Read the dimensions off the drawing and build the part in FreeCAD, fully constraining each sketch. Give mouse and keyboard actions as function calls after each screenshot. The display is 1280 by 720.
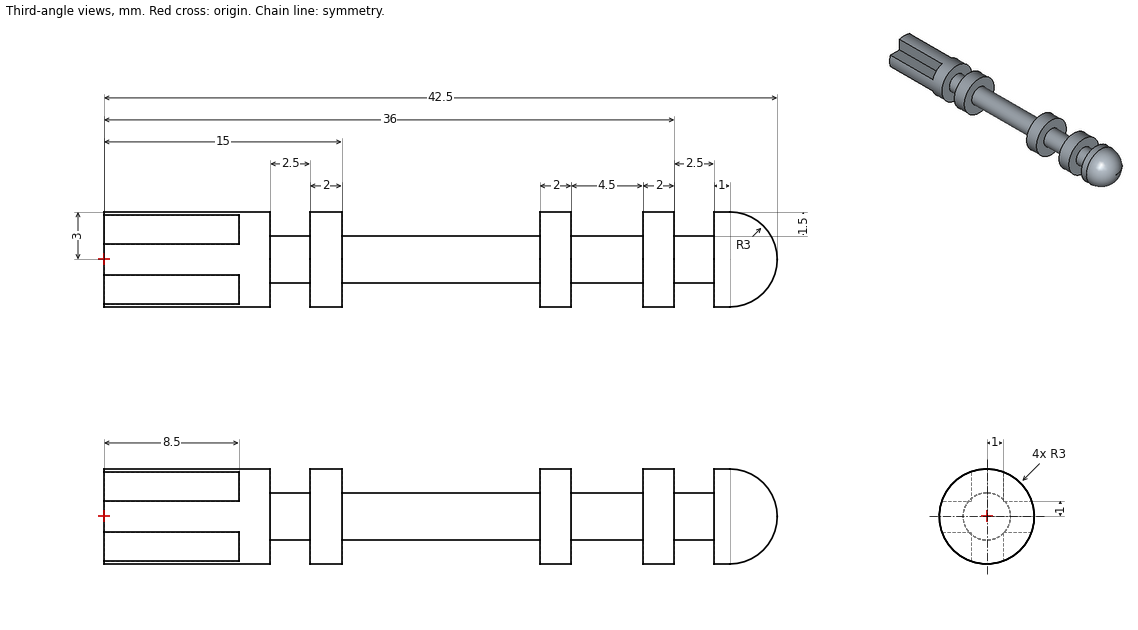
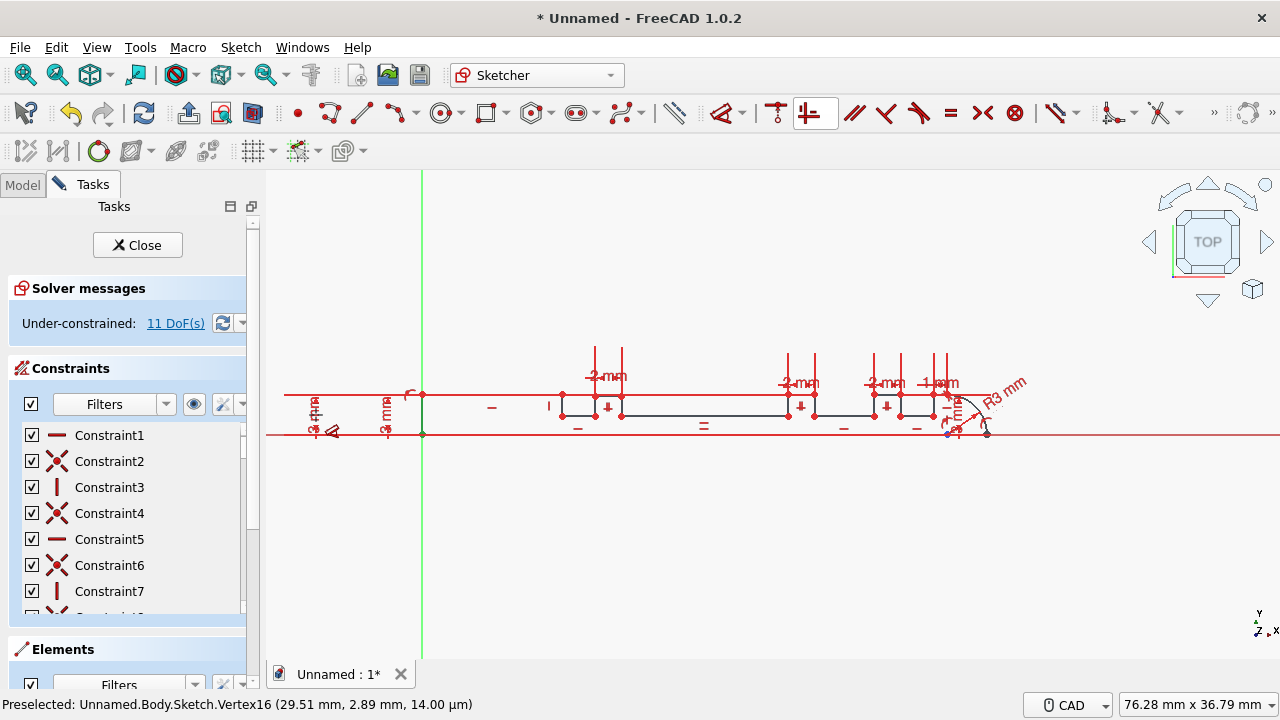
click(622, 396)
click(656, 402)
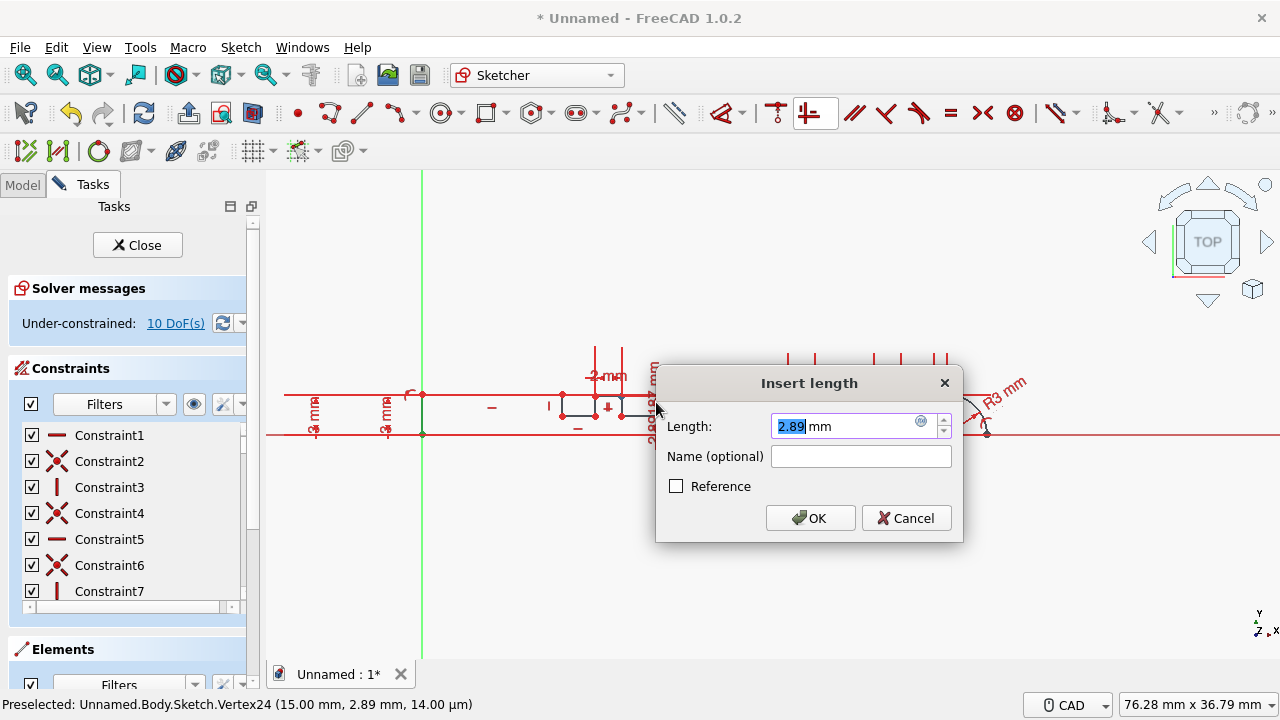
text(3)
key(Return)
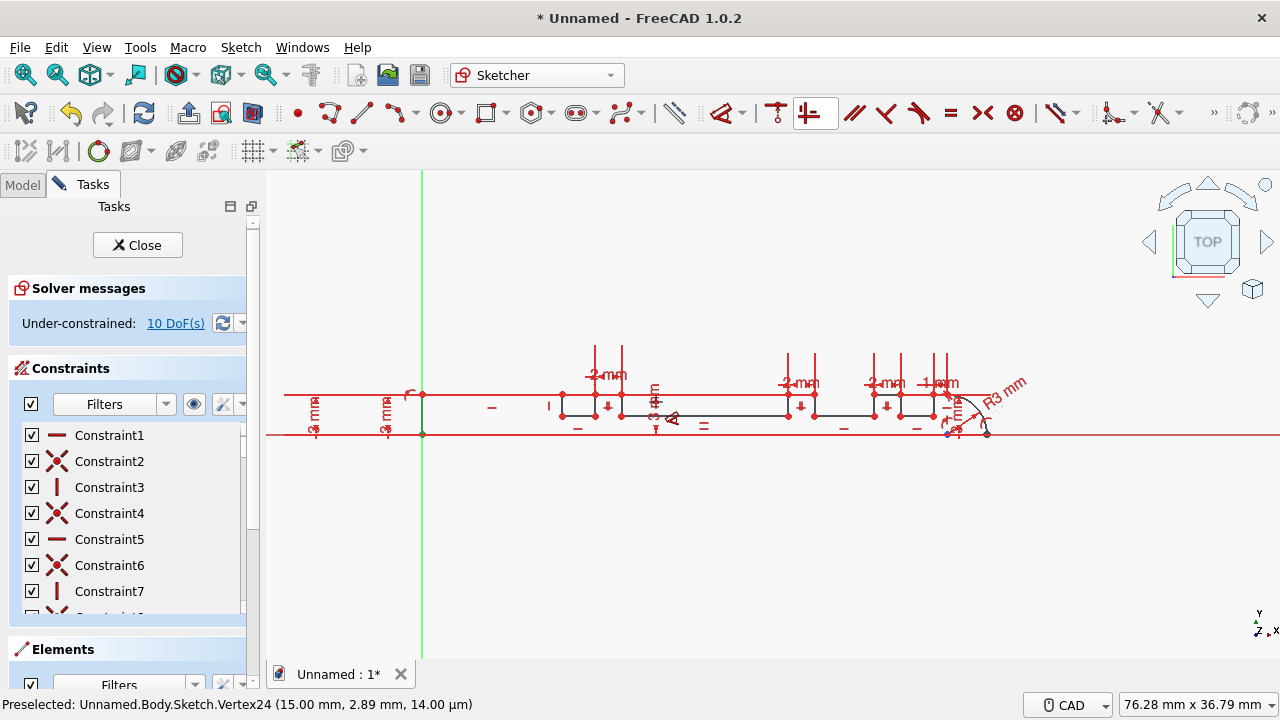
scroll(934, 406, up, 4)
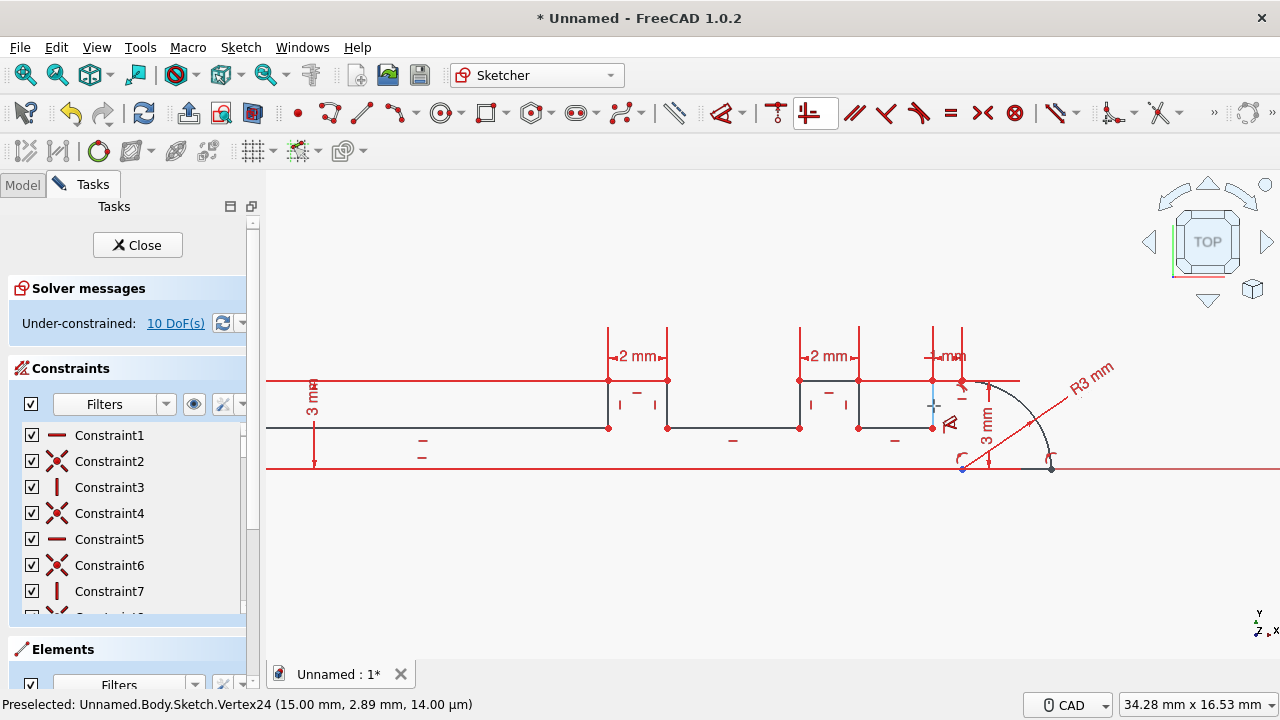
click(933, 404)
click(967, 404)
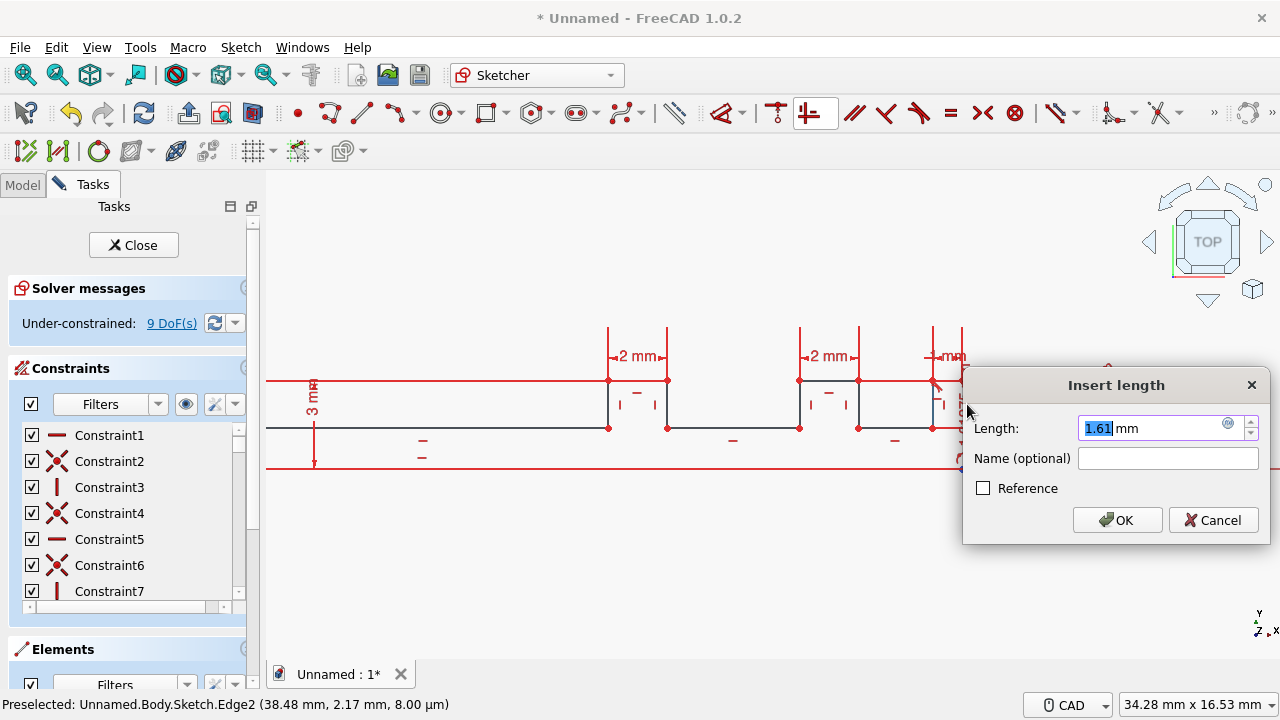
text(1.5)
key(Return)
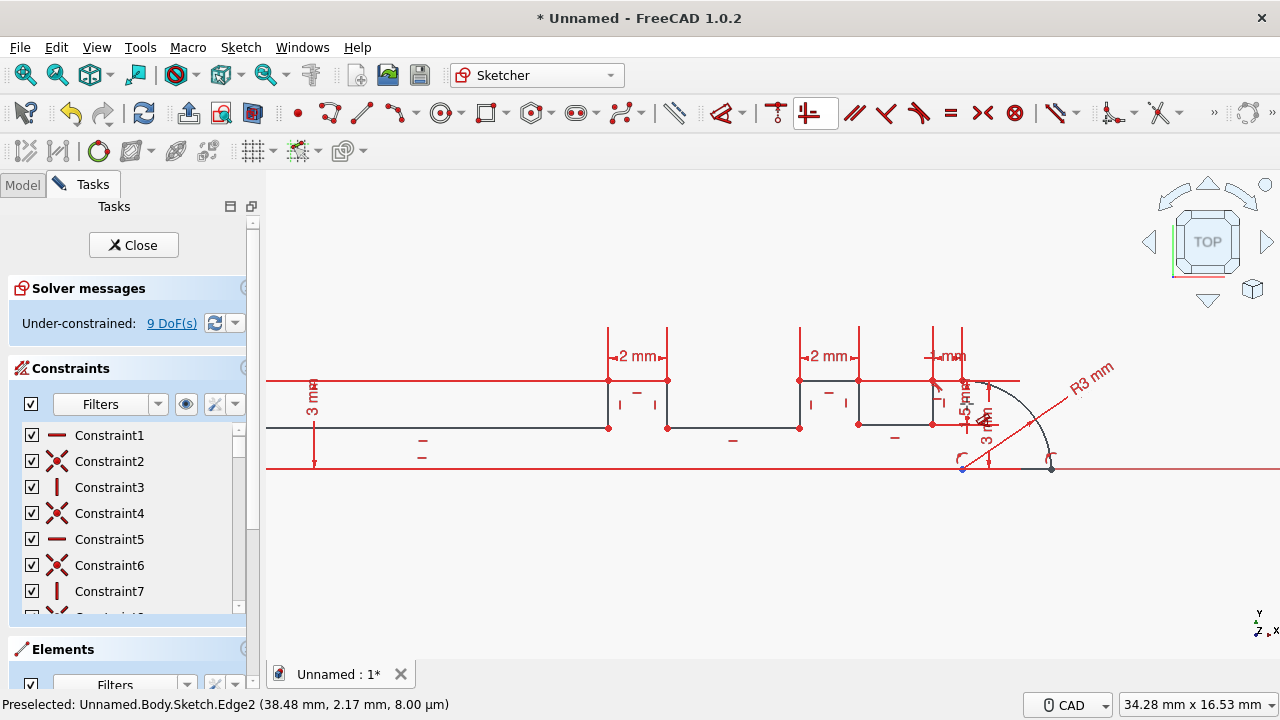
click(911, 425)
click(896, 391)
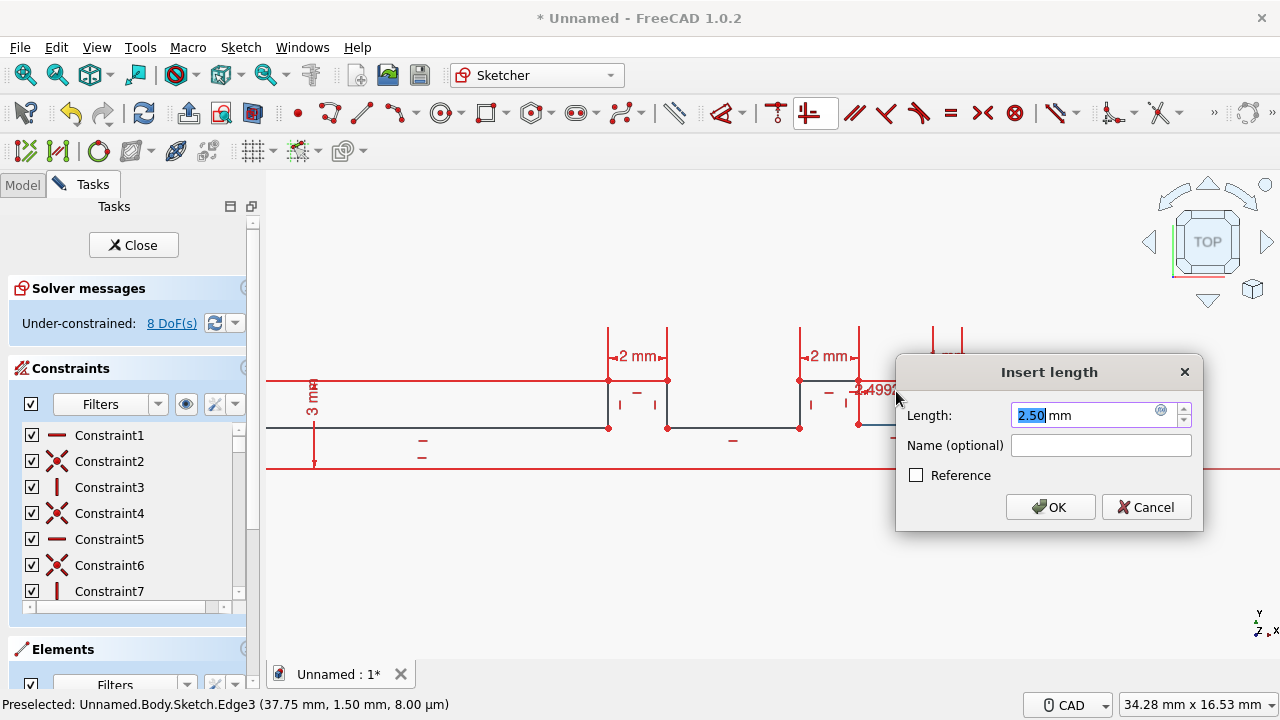
text(2.5)
key(Return)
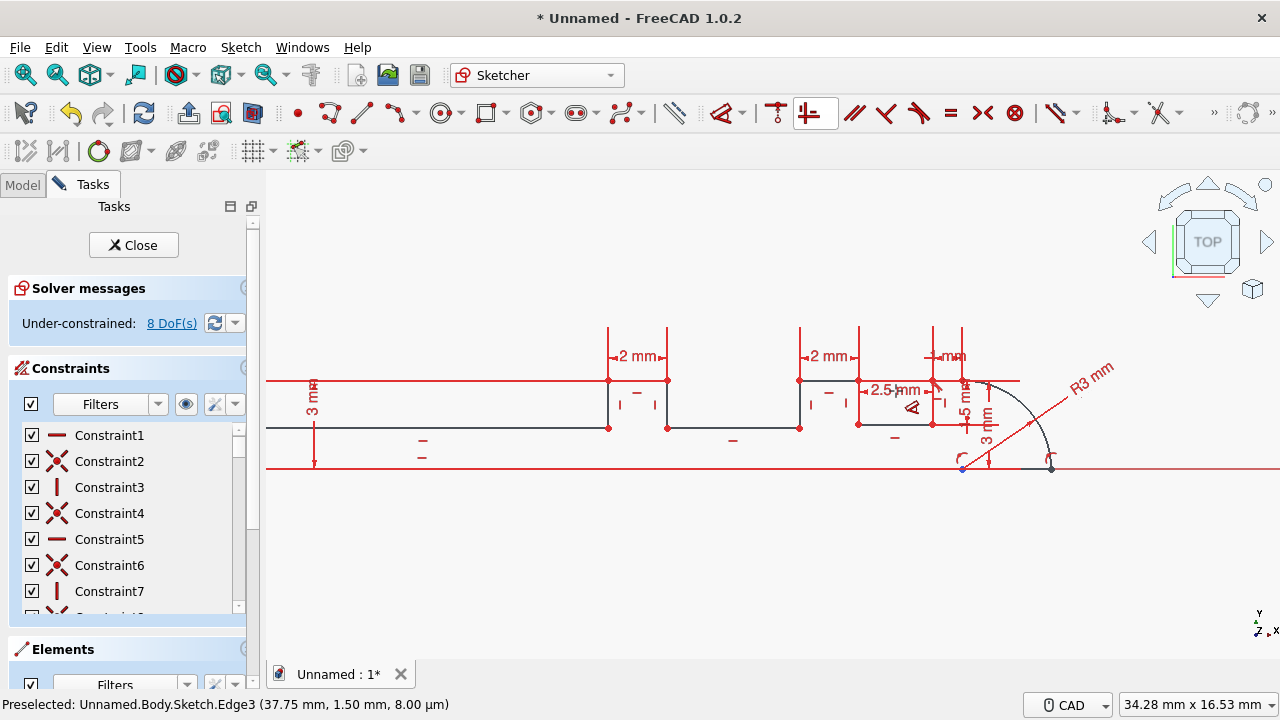
click(800, 395)
click(834, 415)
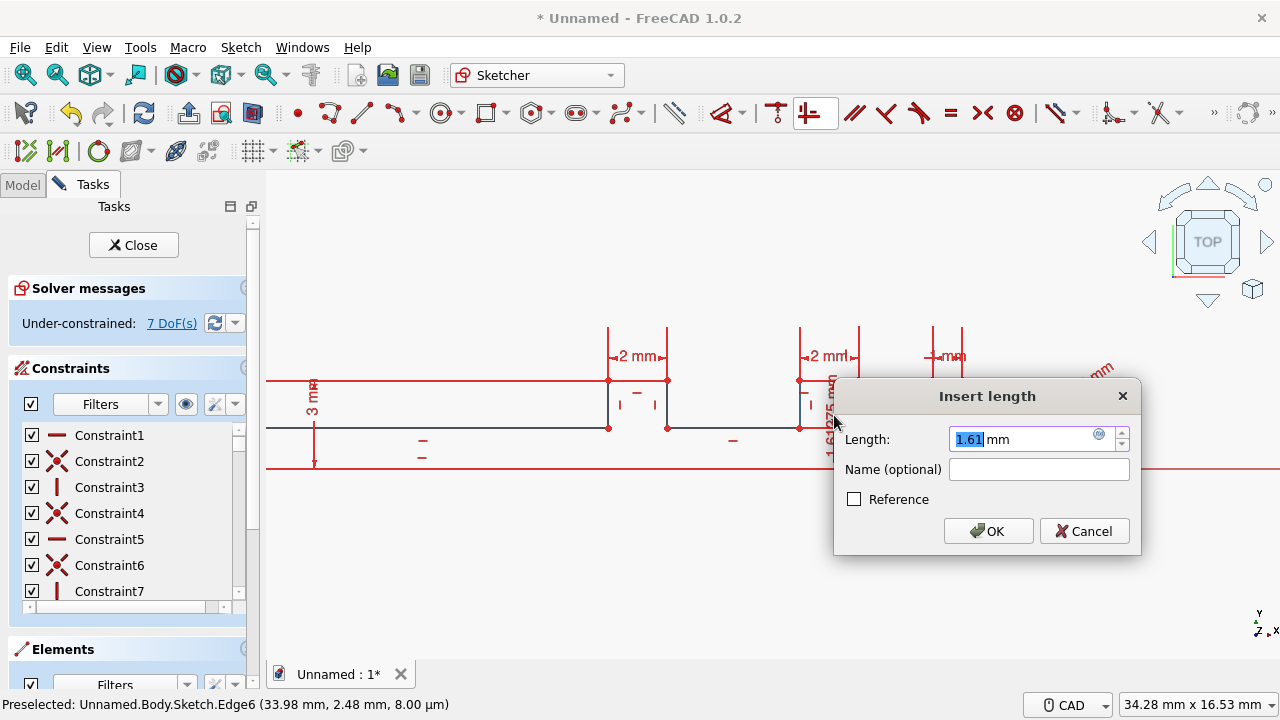
text(1.5)
key(Return)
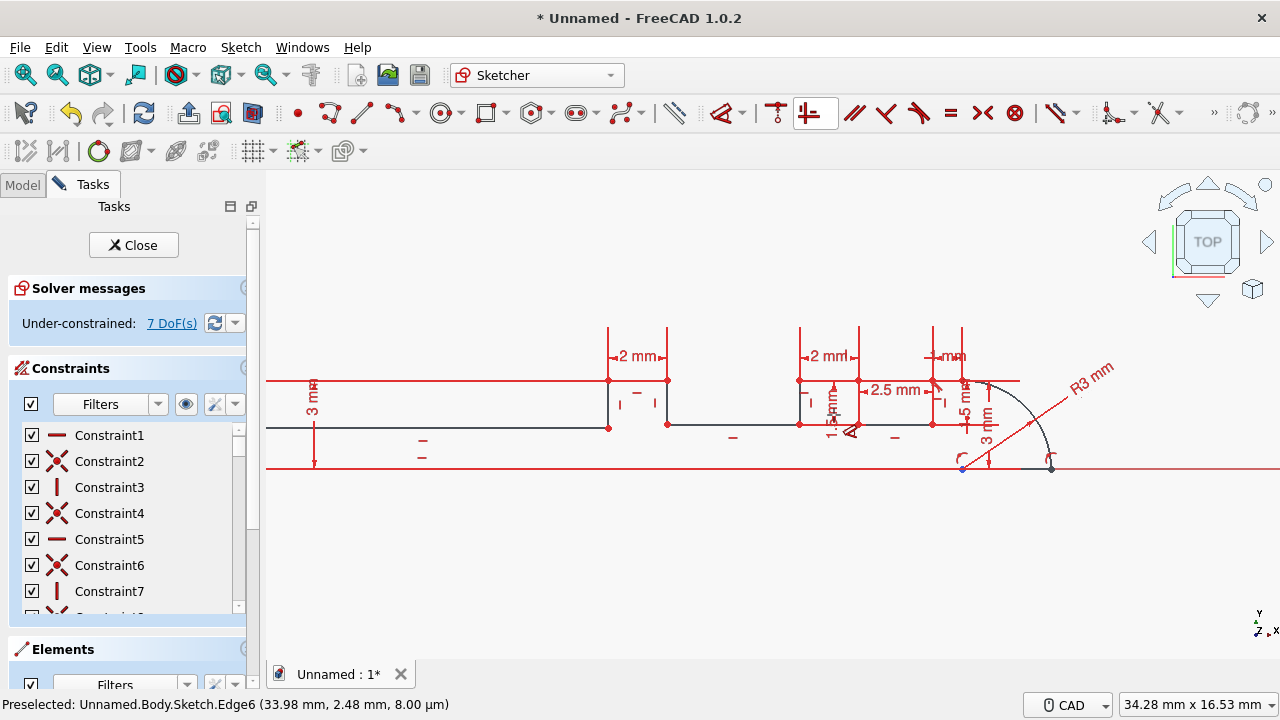
click(760, 425)
click(734, 391)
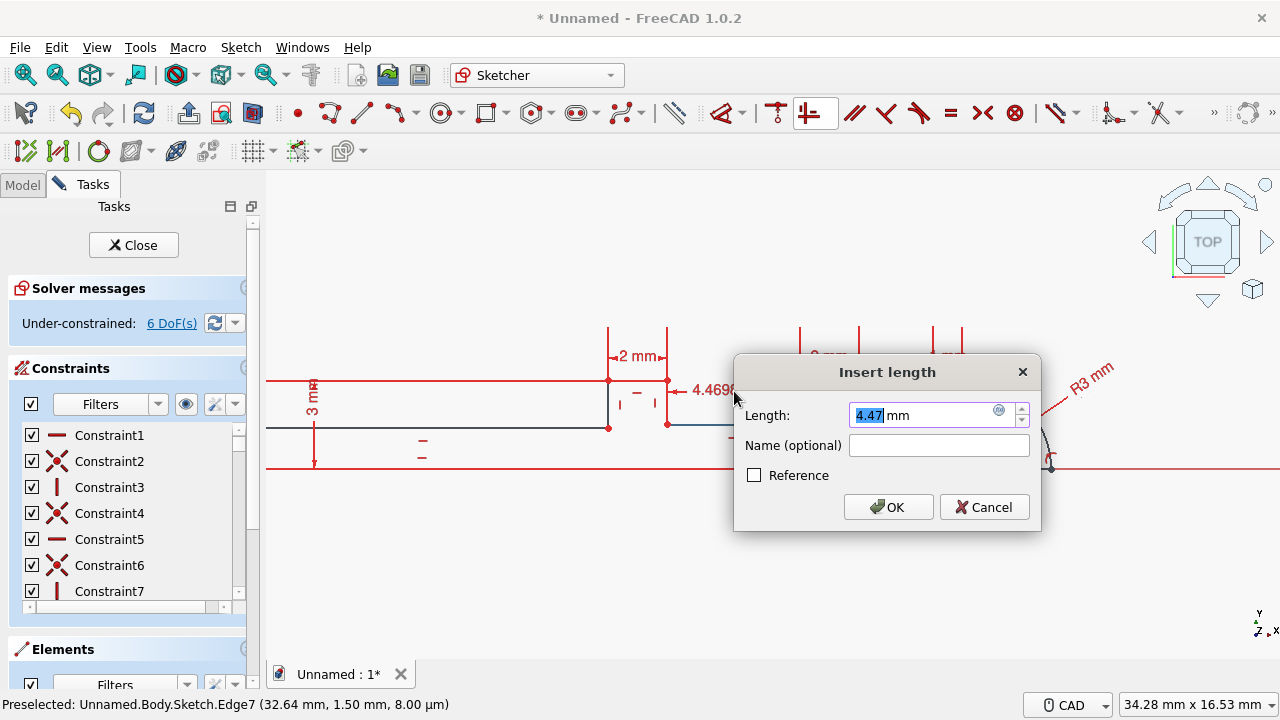
text(4.5)
key(Return)